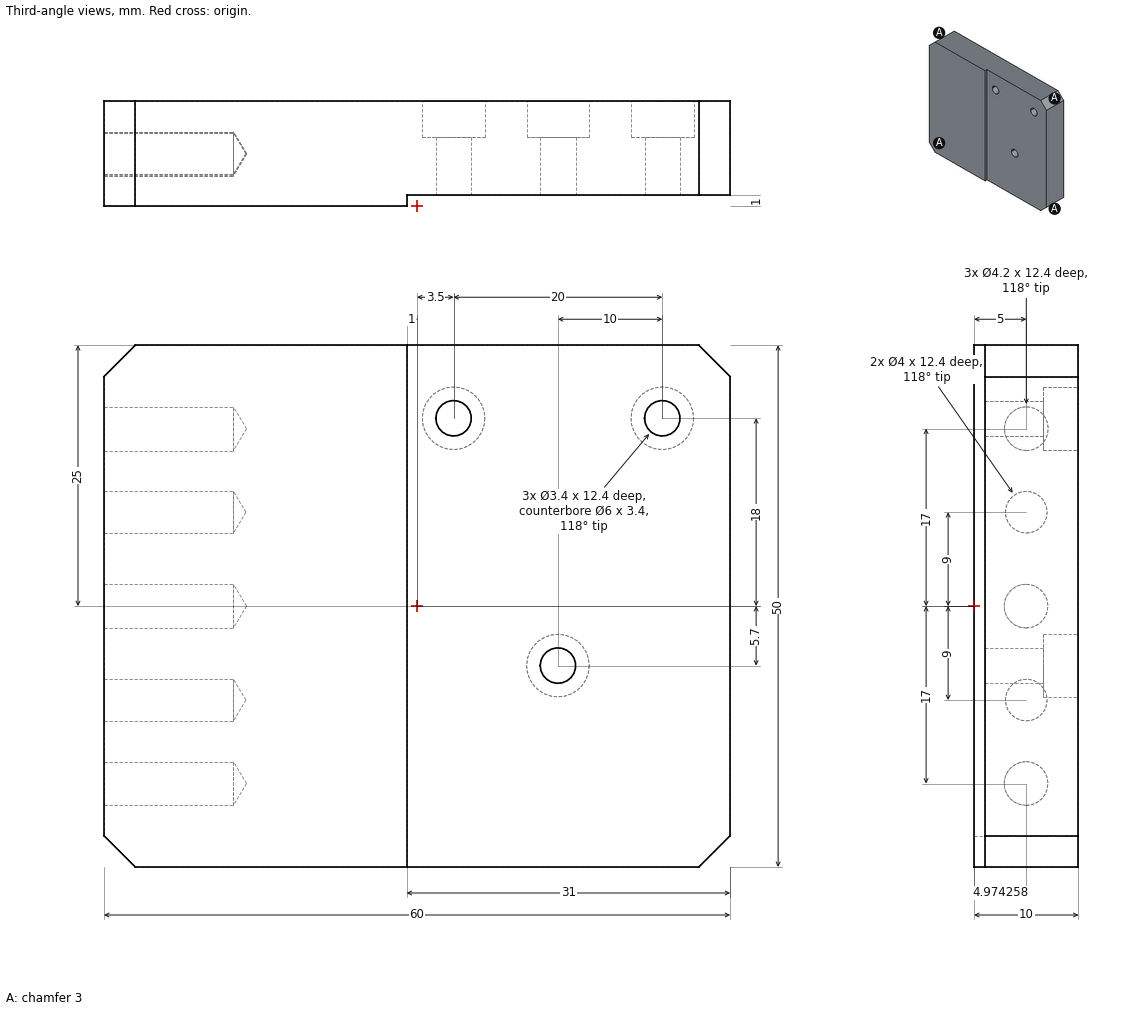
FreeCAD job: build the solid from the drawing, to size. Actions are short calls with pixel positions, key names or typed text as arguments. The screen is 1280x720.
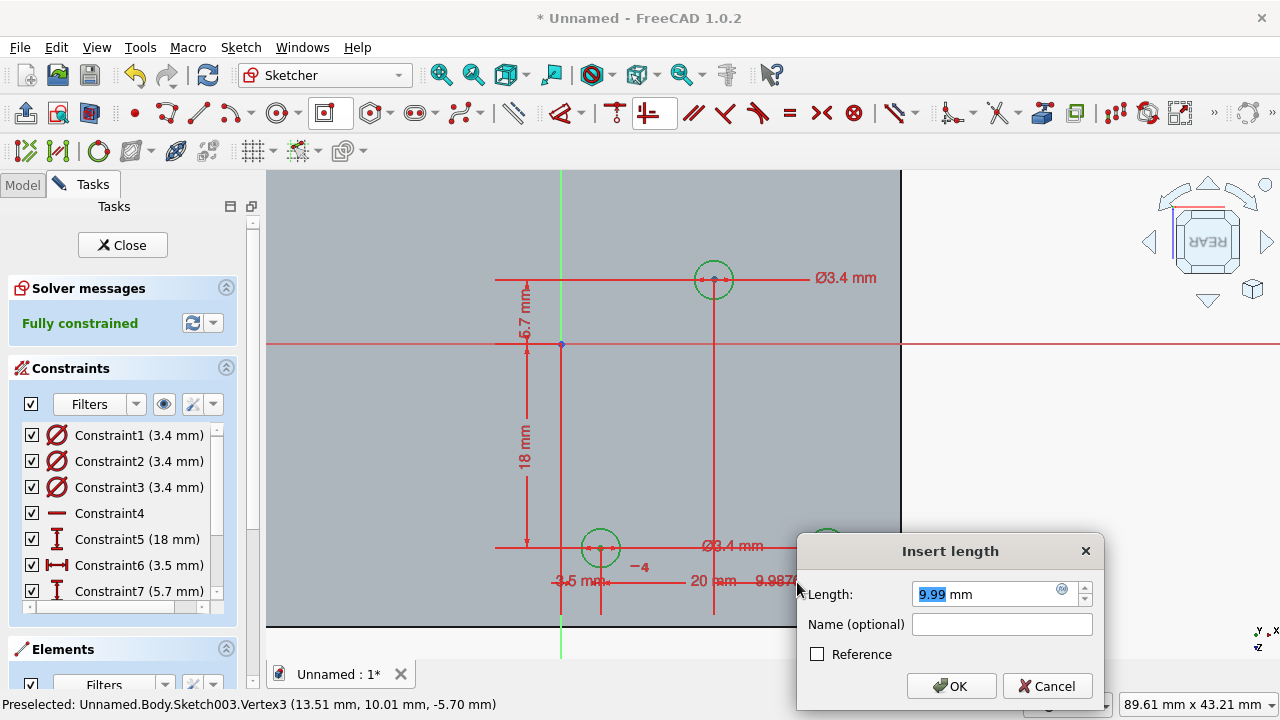
text(10)
key(Return)
key(Escape)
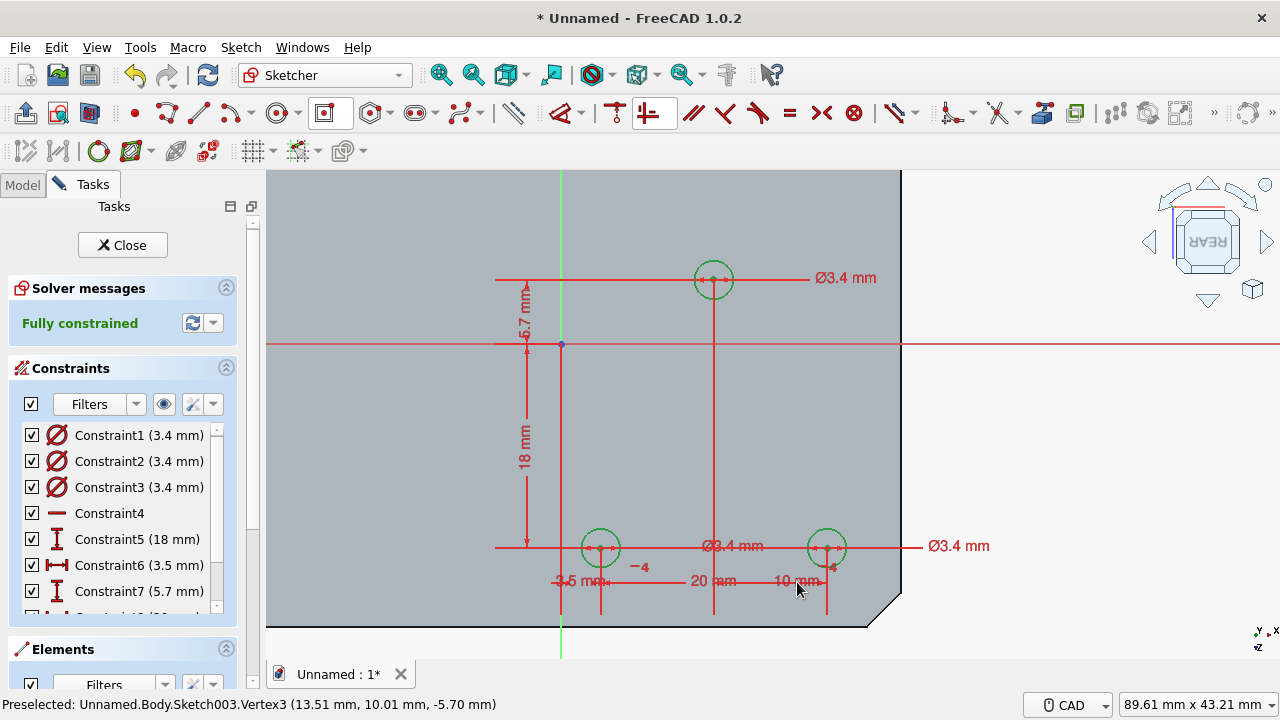
click(123, 245)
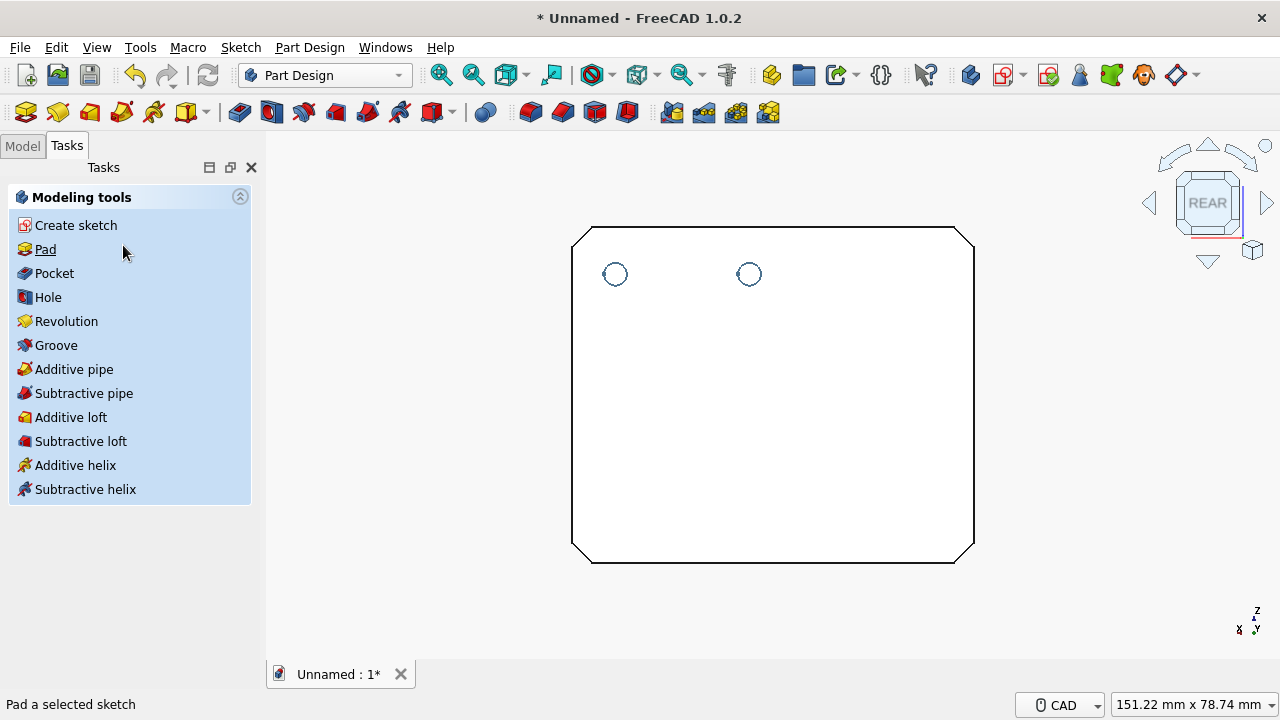
click(272, 112)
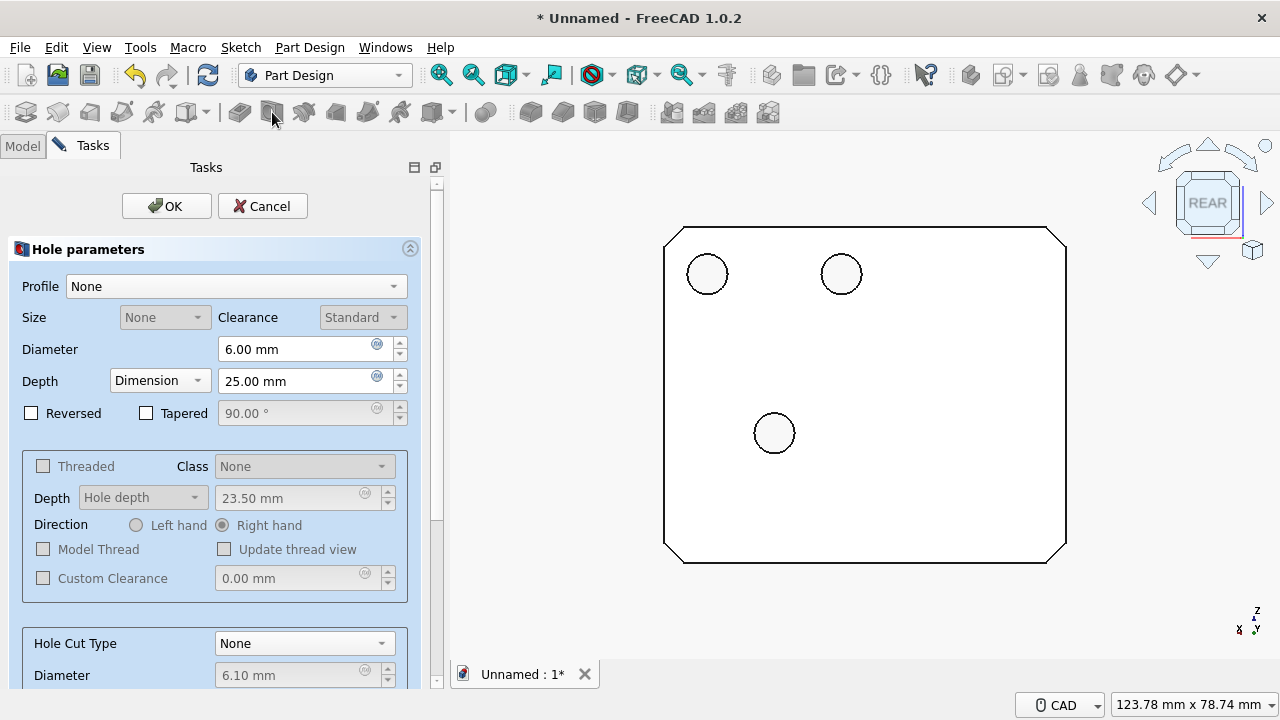
triple_click(305, 349)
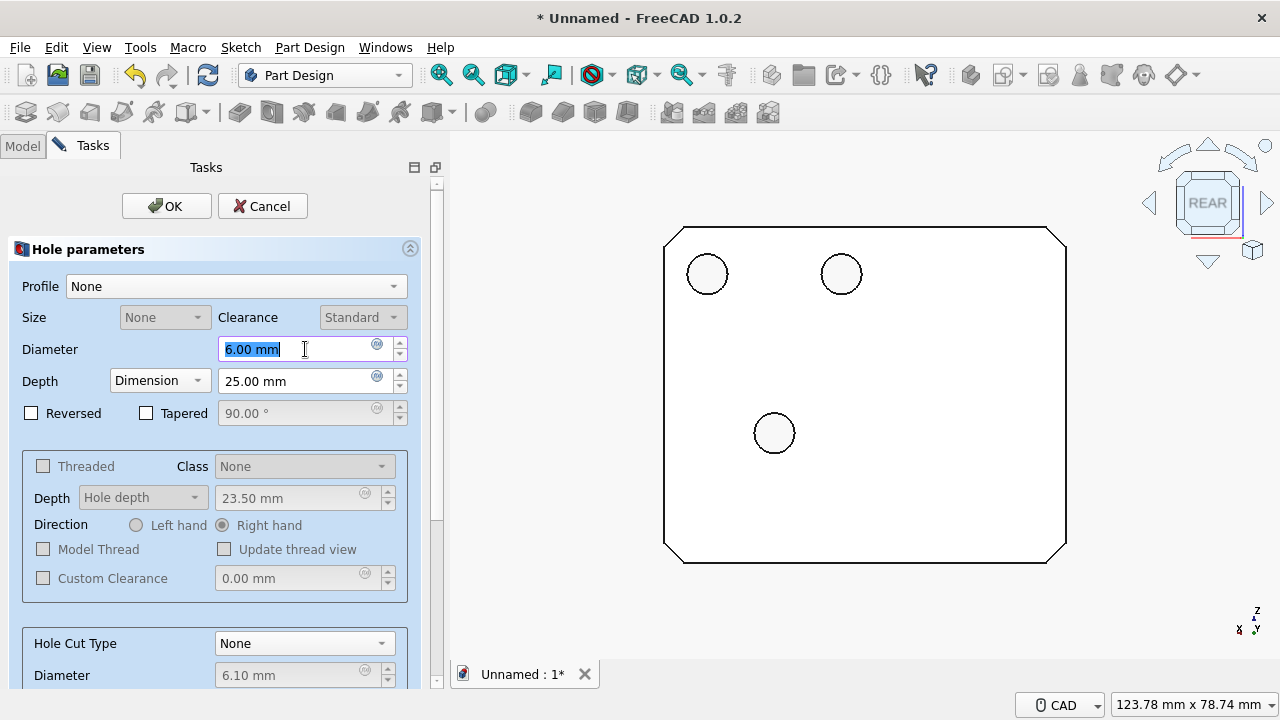
text(3.4)
key(Tab)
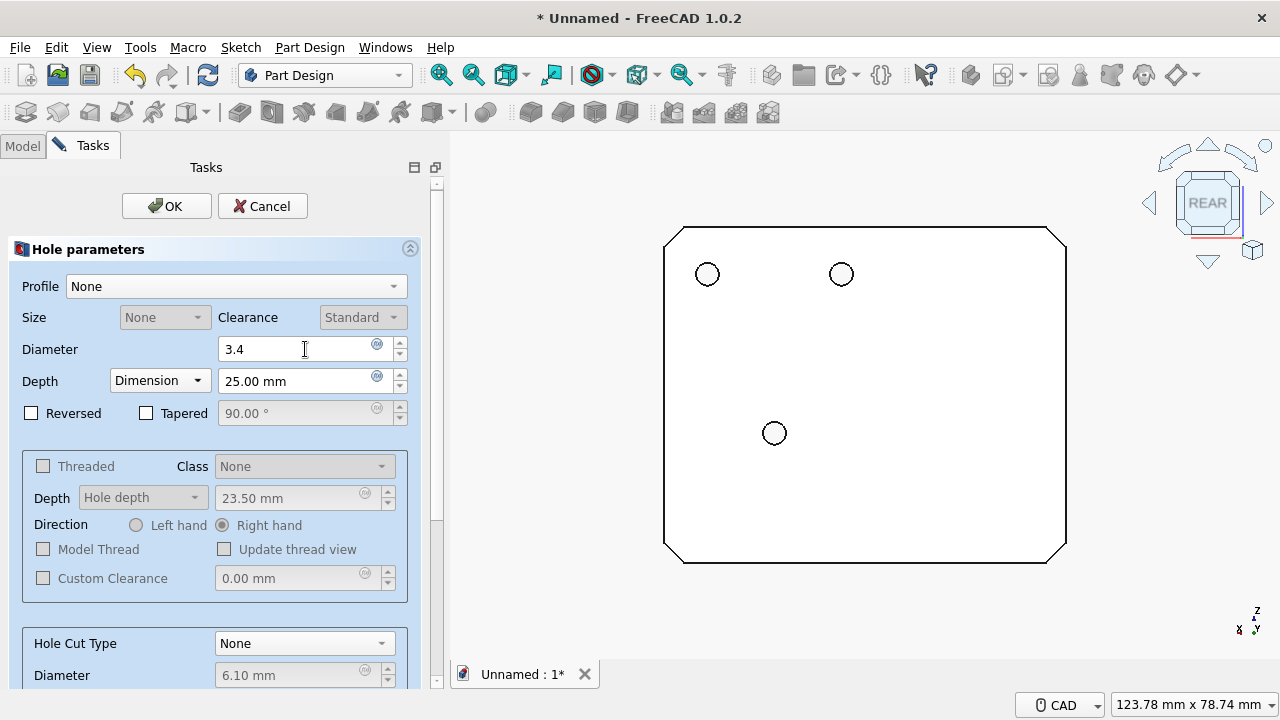
triple_click(305, 381)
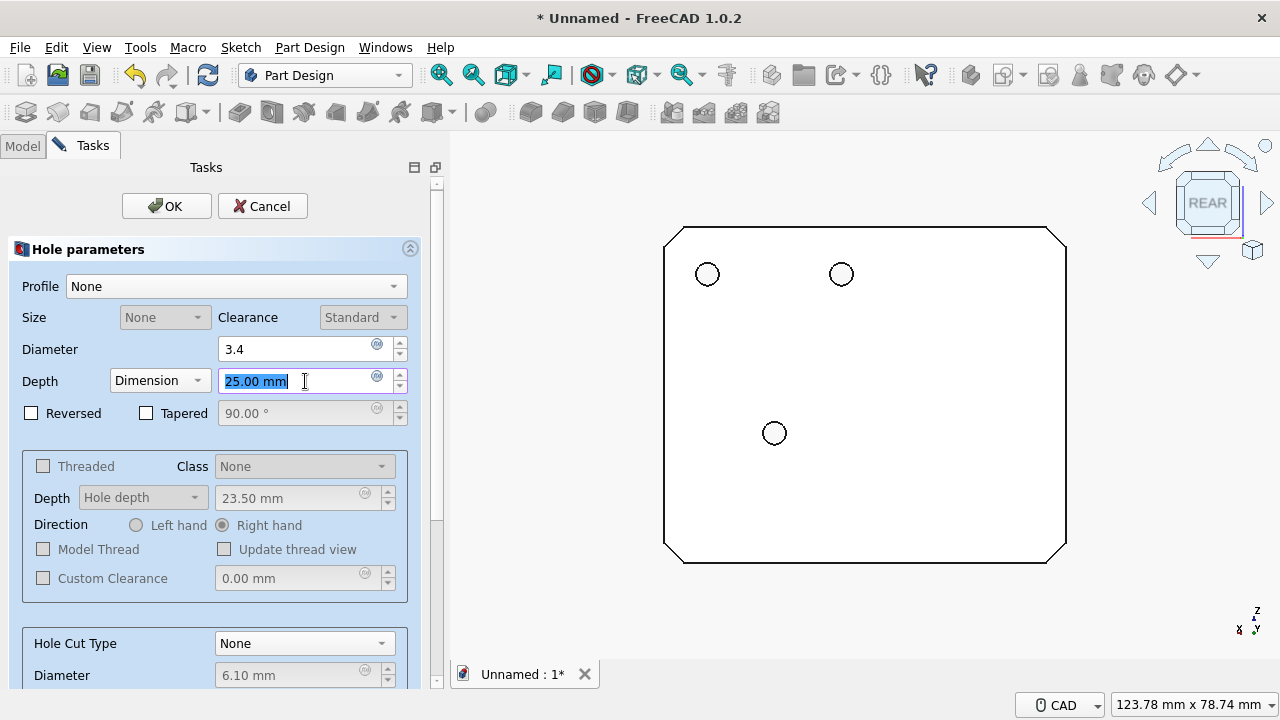
text(12.4)
key(Tab)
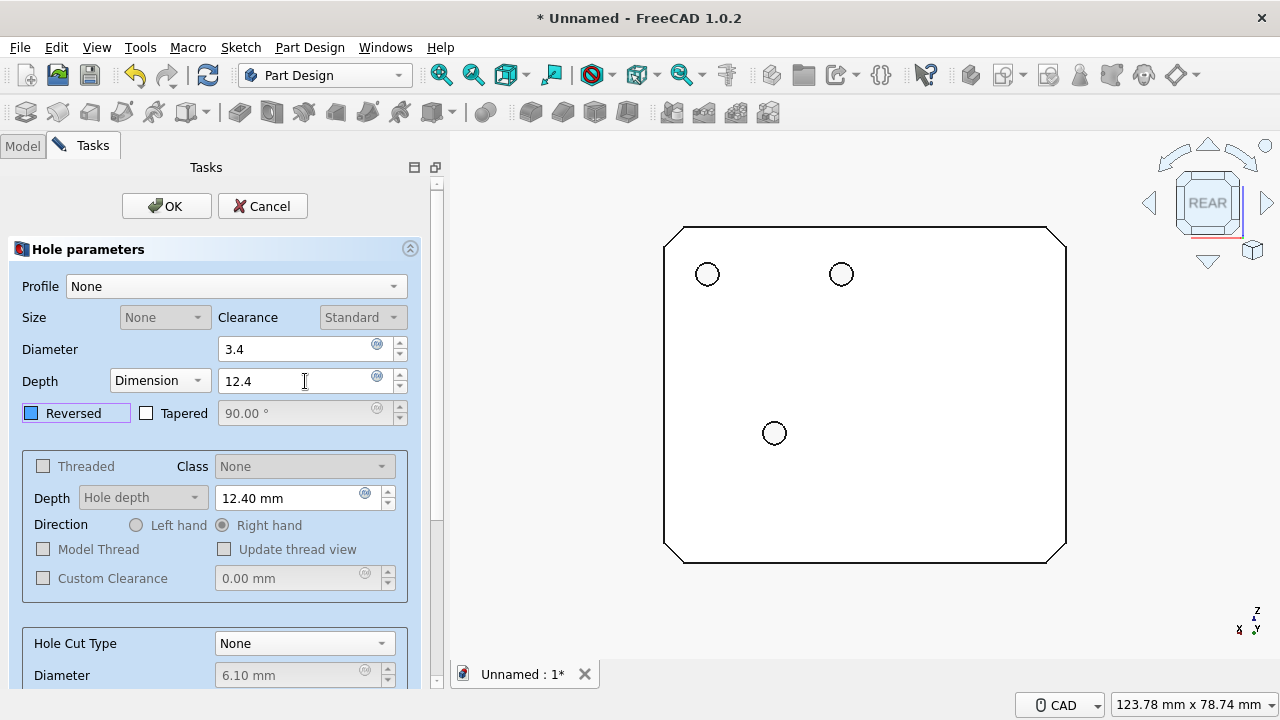
click(306, 644)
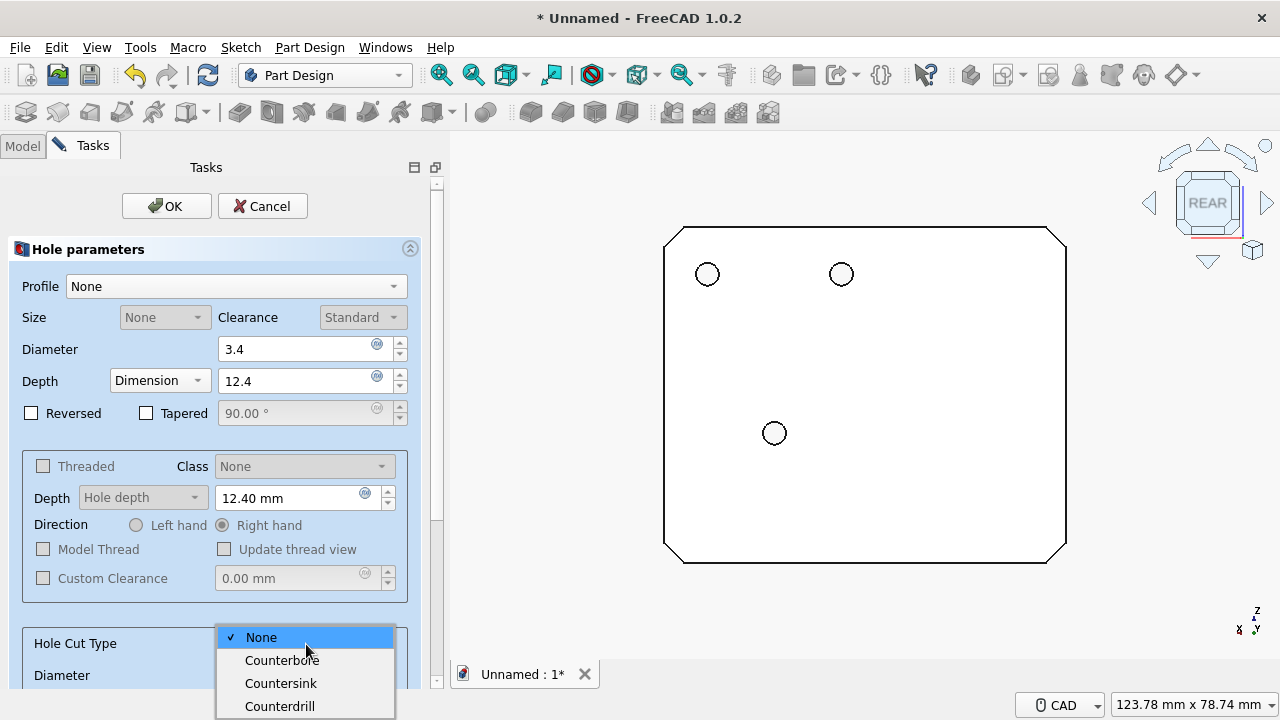
click(304, 660)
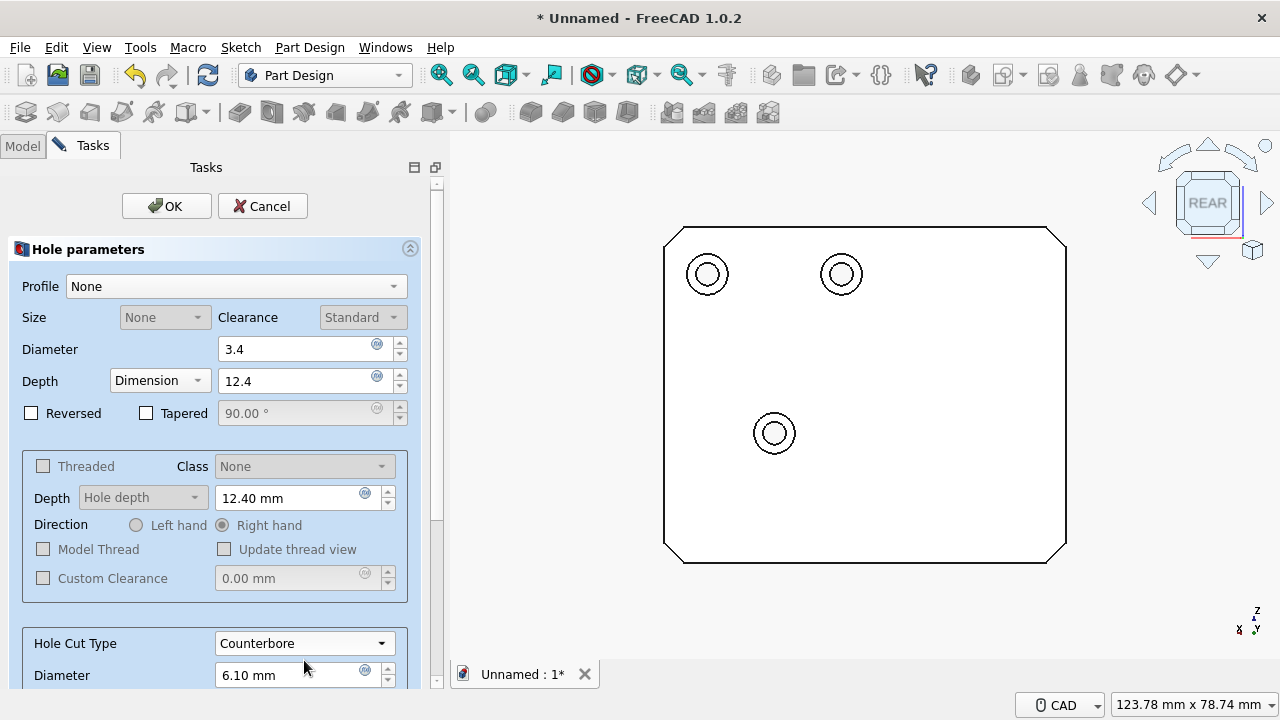
triple_click(298, 675)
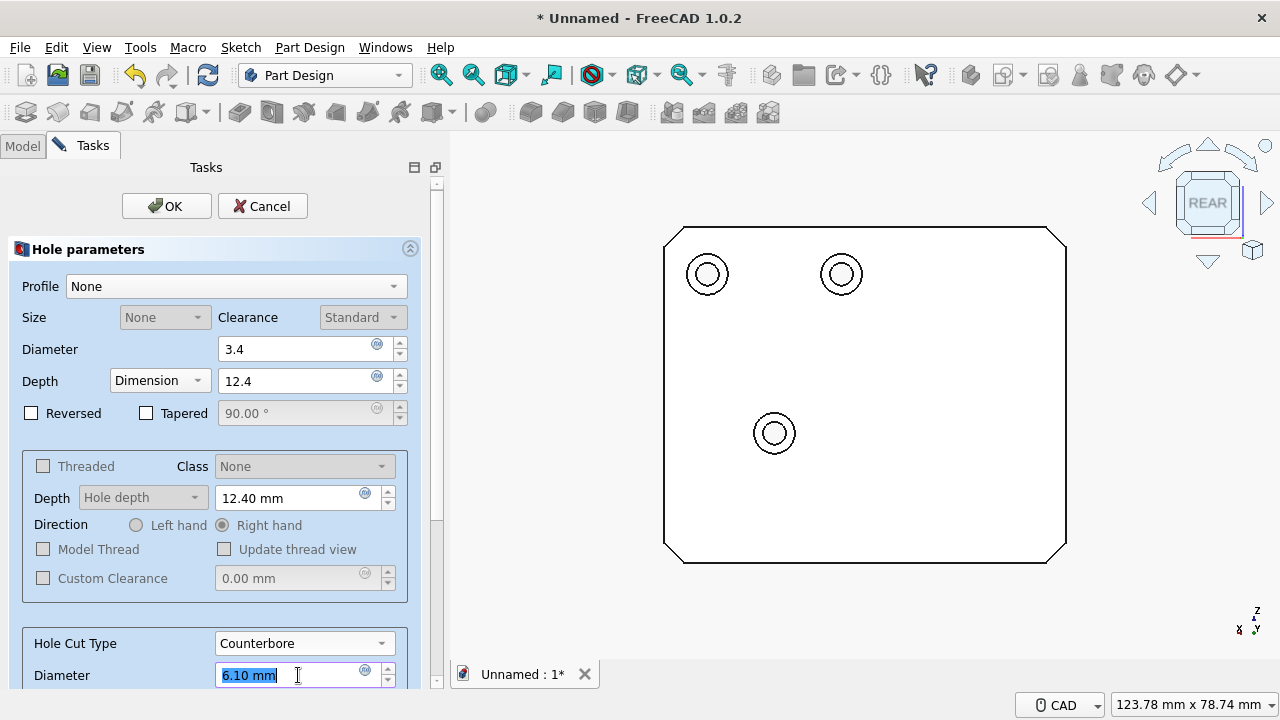
text(6)
key(Tab)